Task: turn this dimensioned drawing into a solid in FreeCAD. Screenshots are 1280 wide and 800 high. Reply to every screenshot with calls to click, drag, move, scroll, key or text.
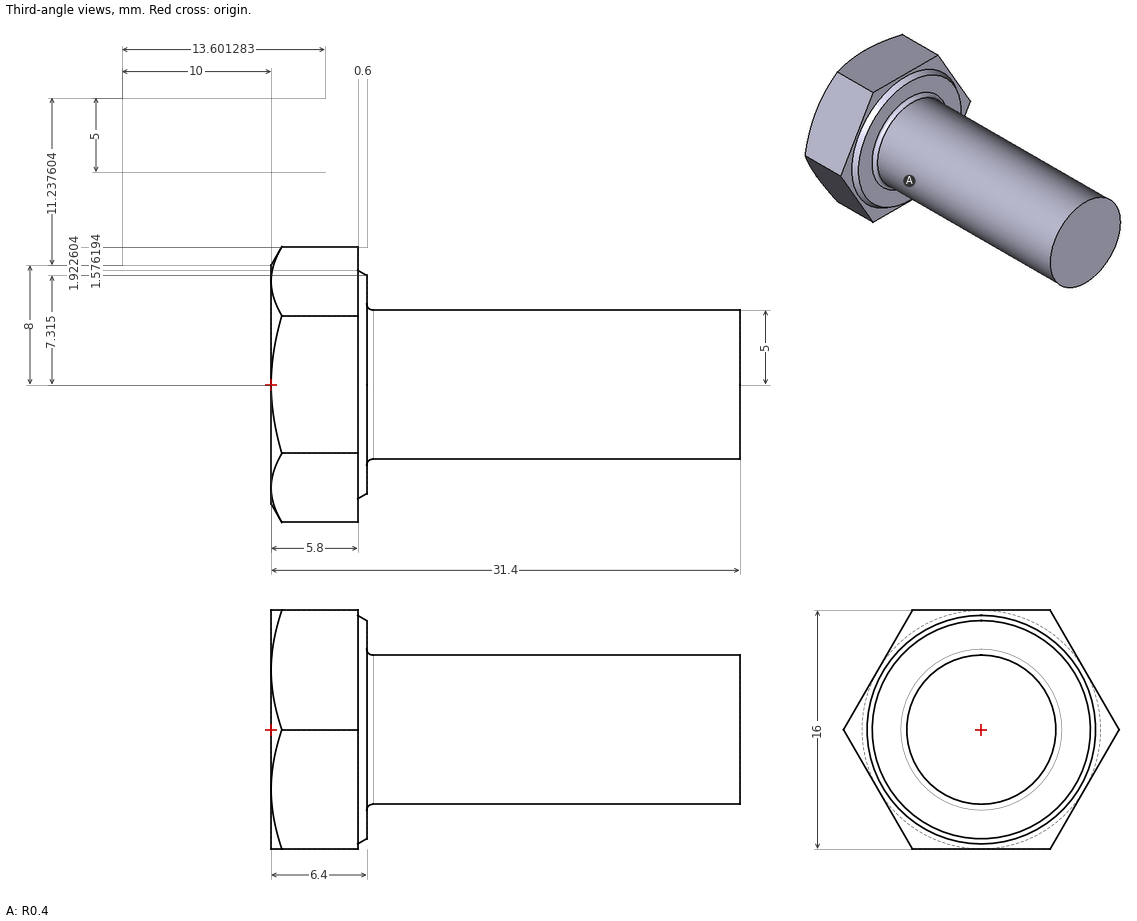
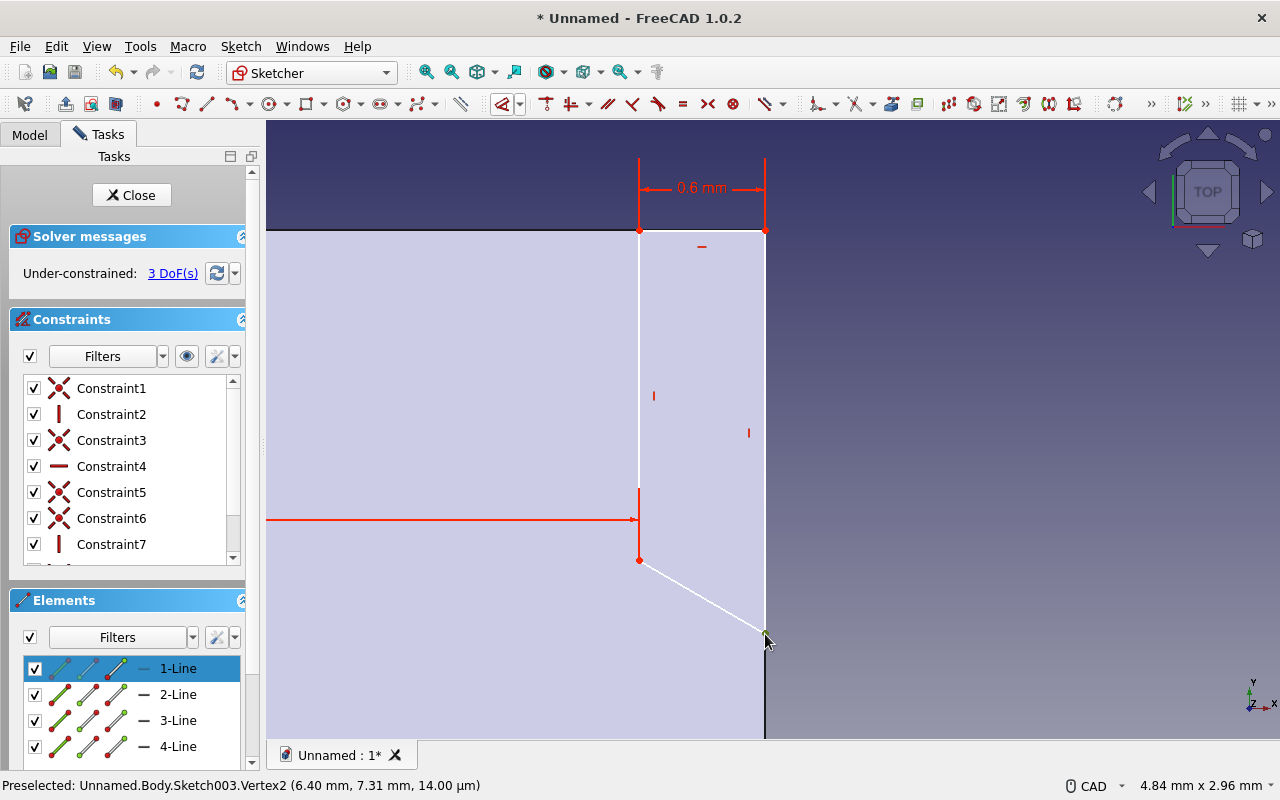
key(i)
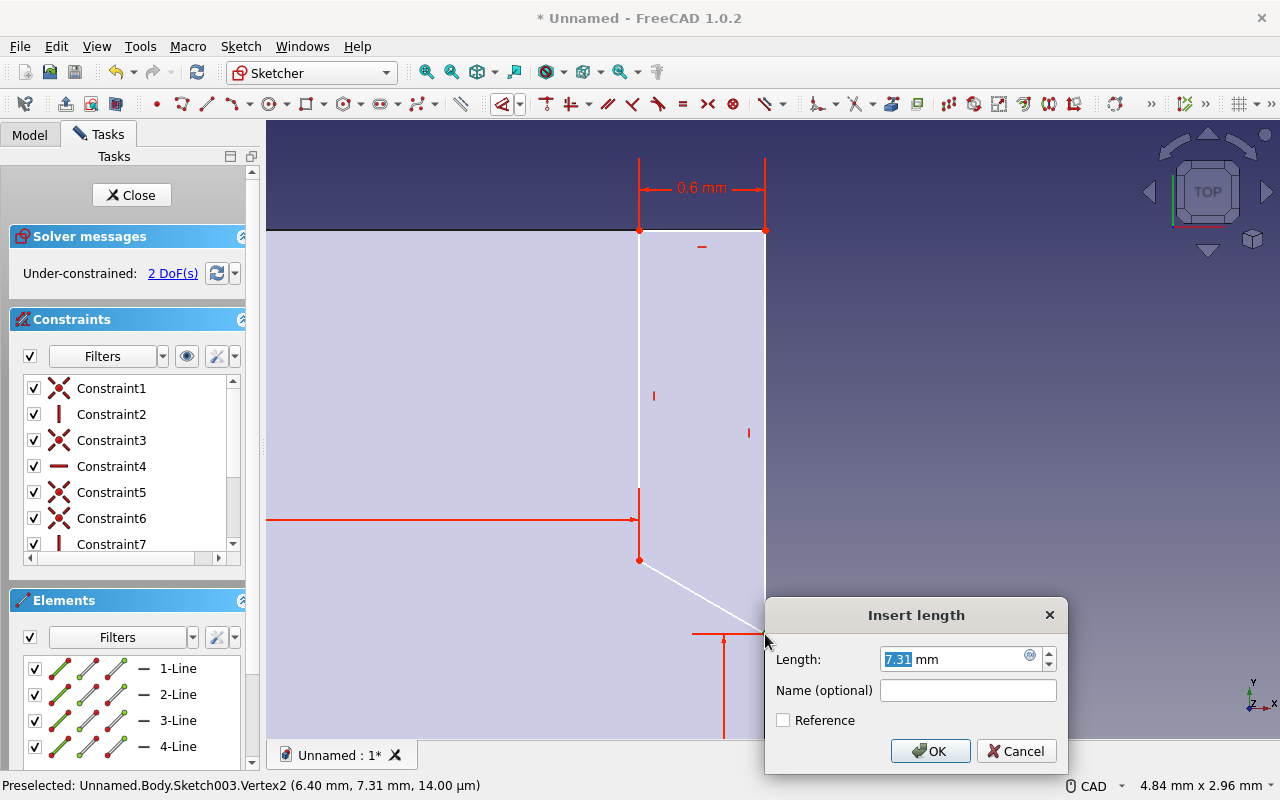
text(7.315)
key(Return)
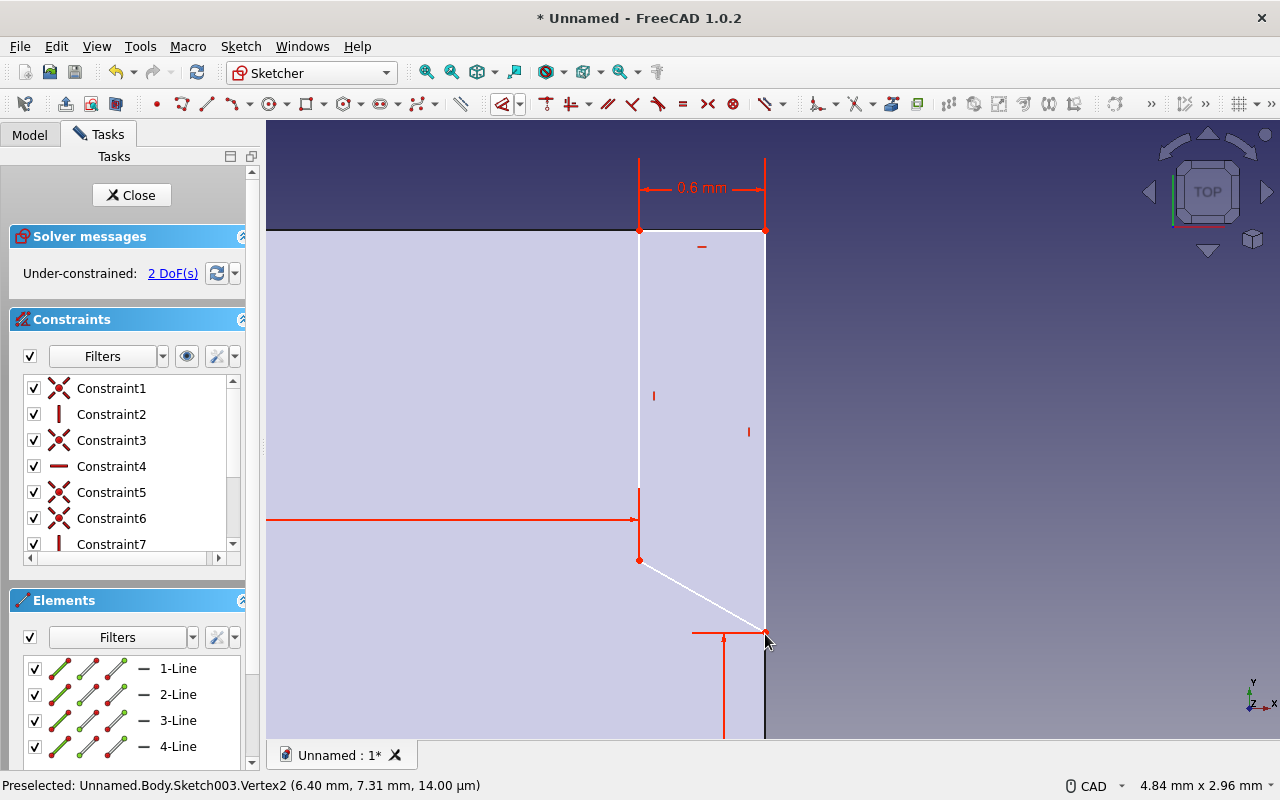
click(765, 512)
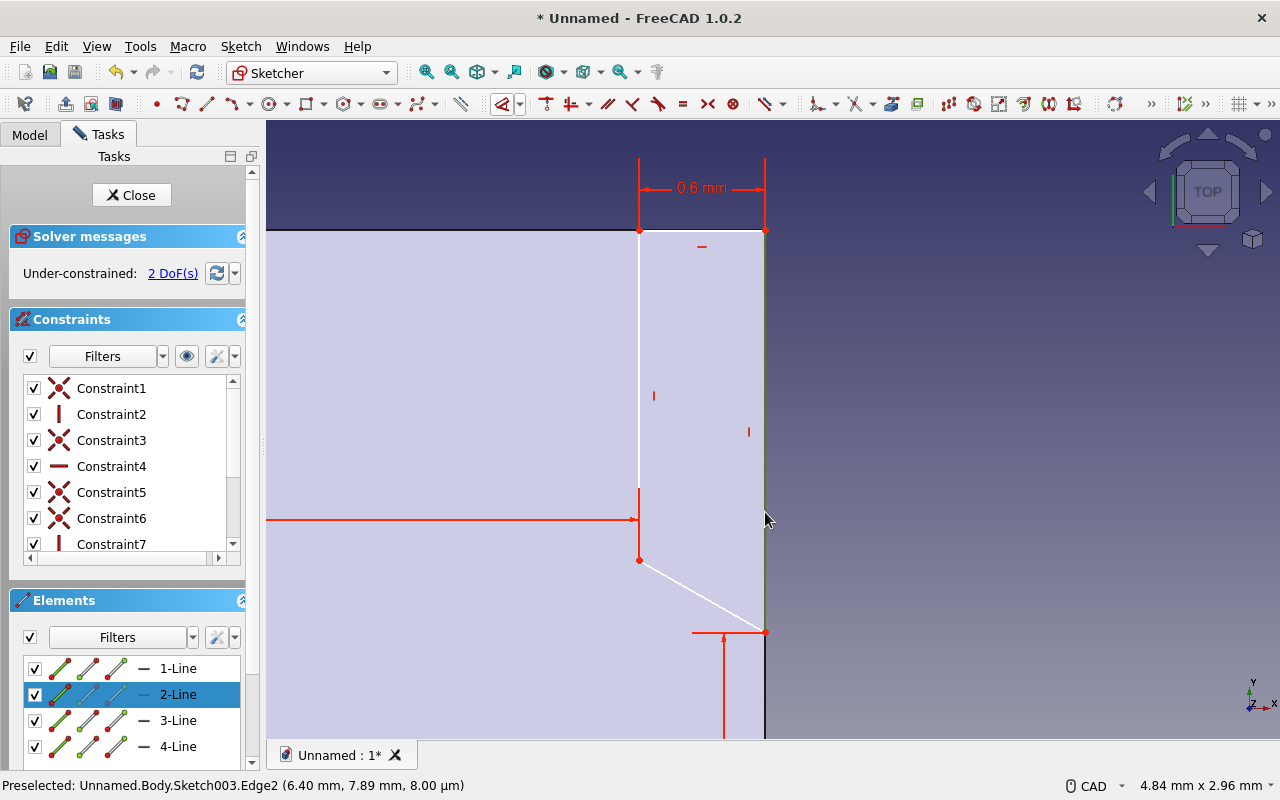
key(i)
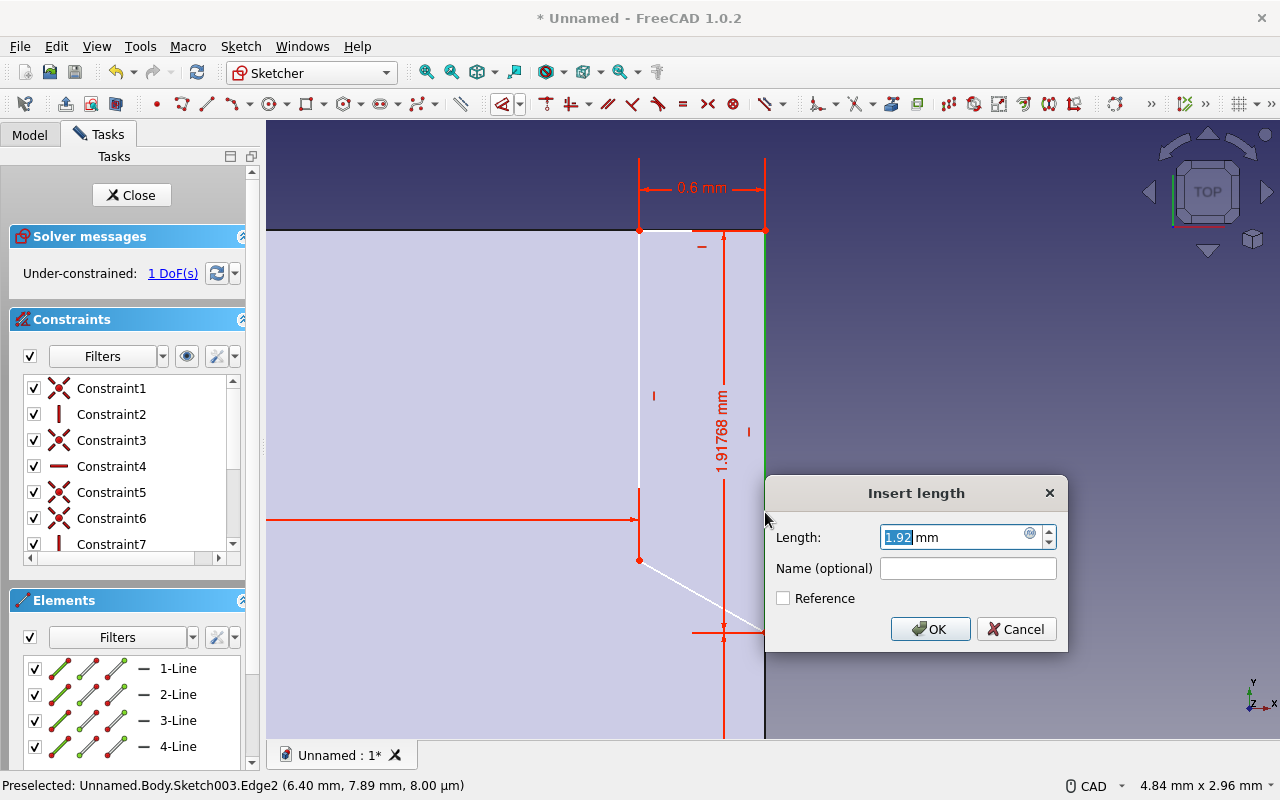
text(1.922604)
key(Return)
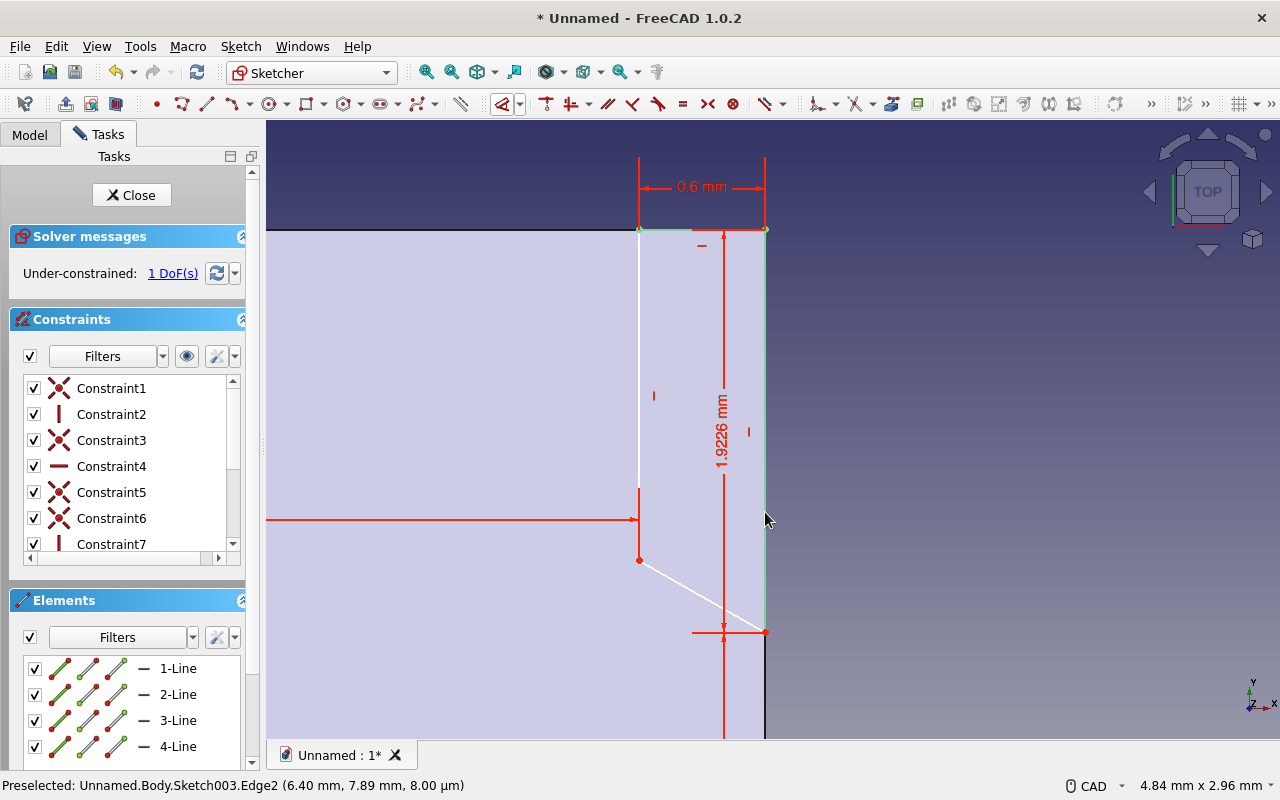
click(639, 329)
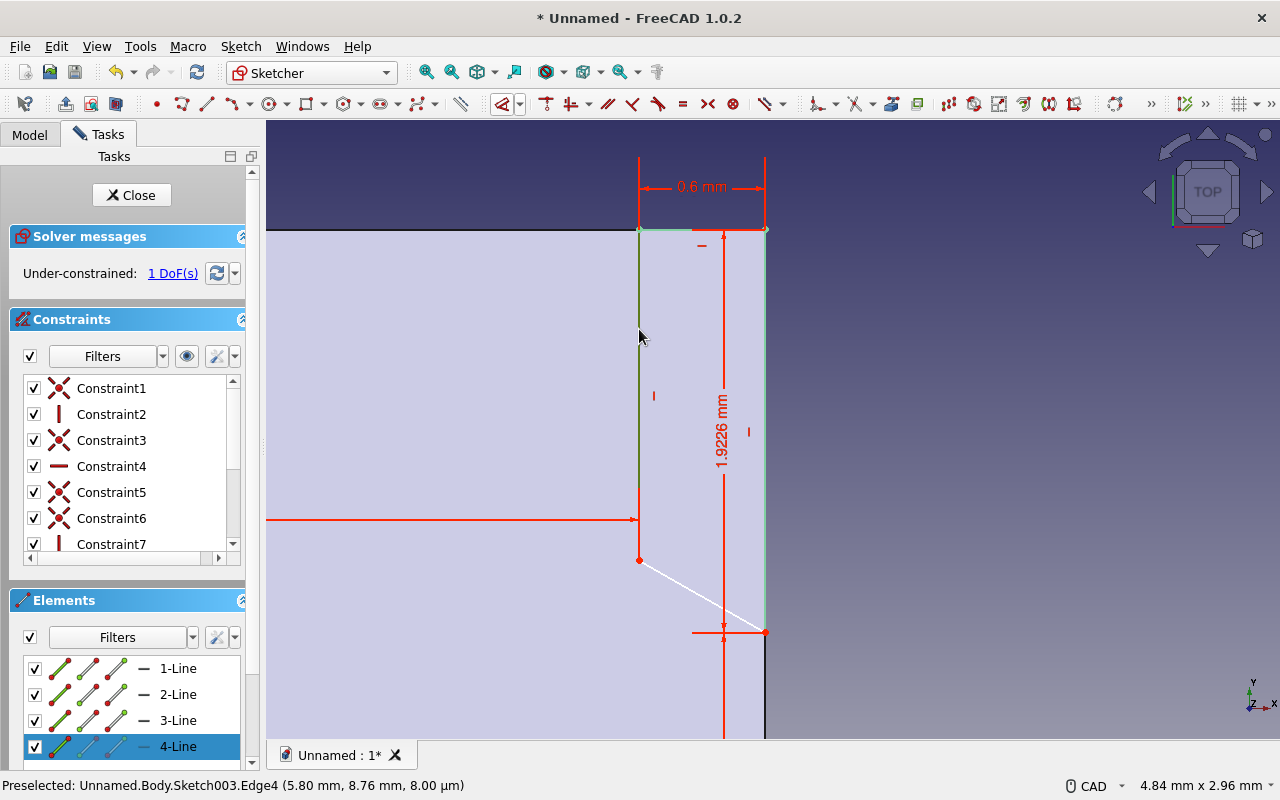
key(i)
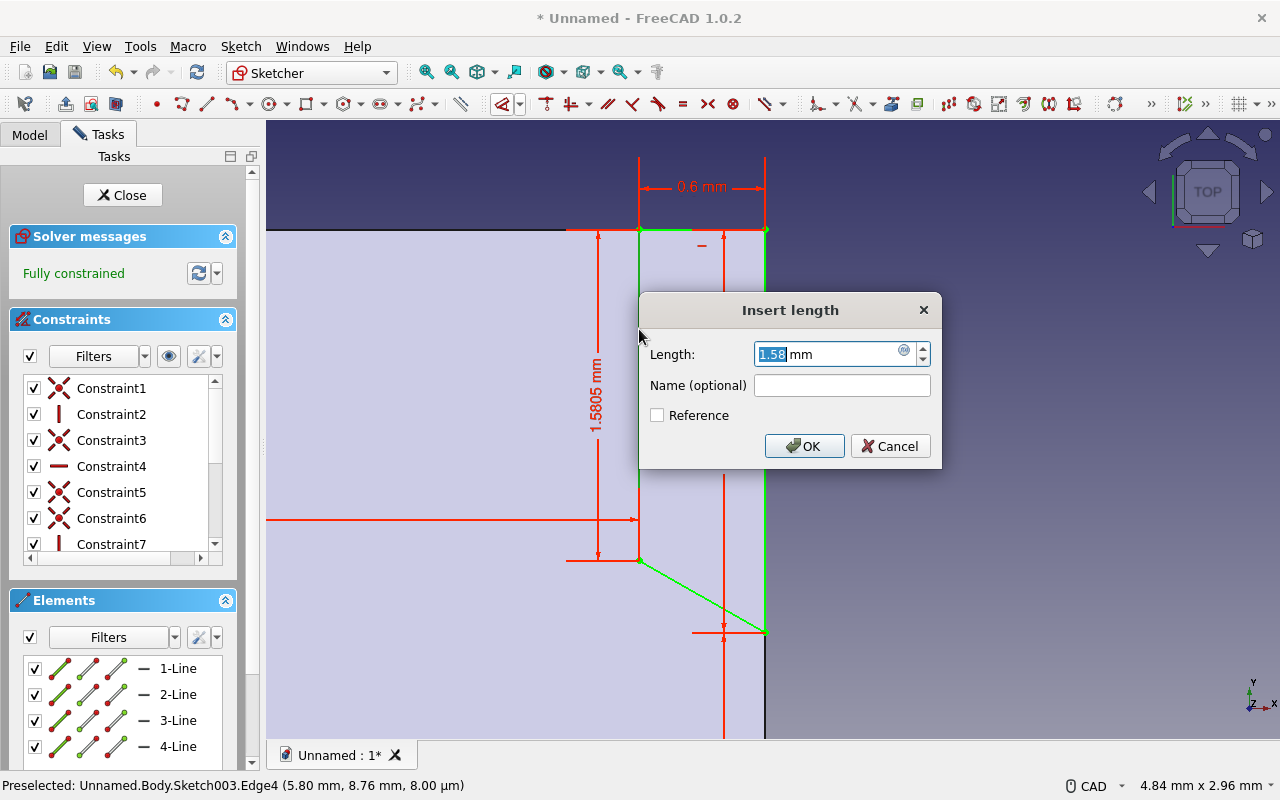
text(1.576194)
key(Return)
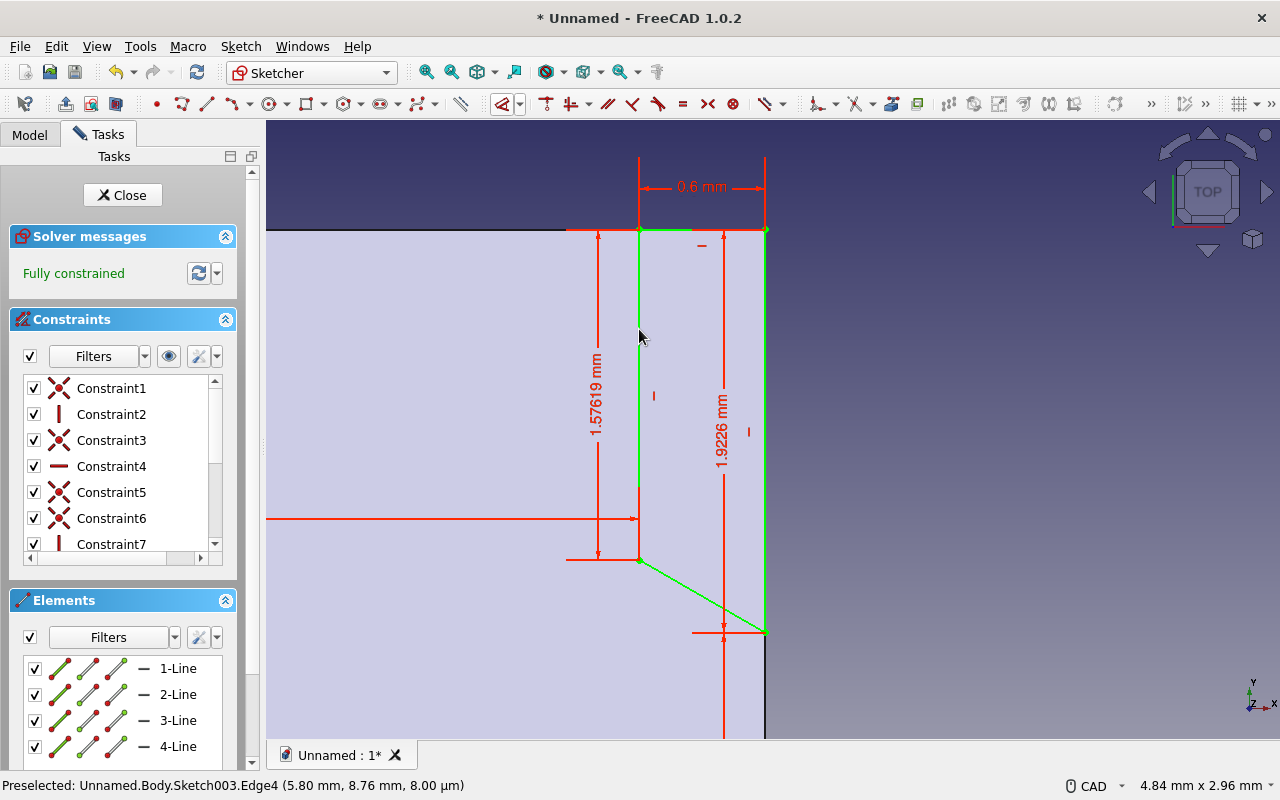
click(123, 195)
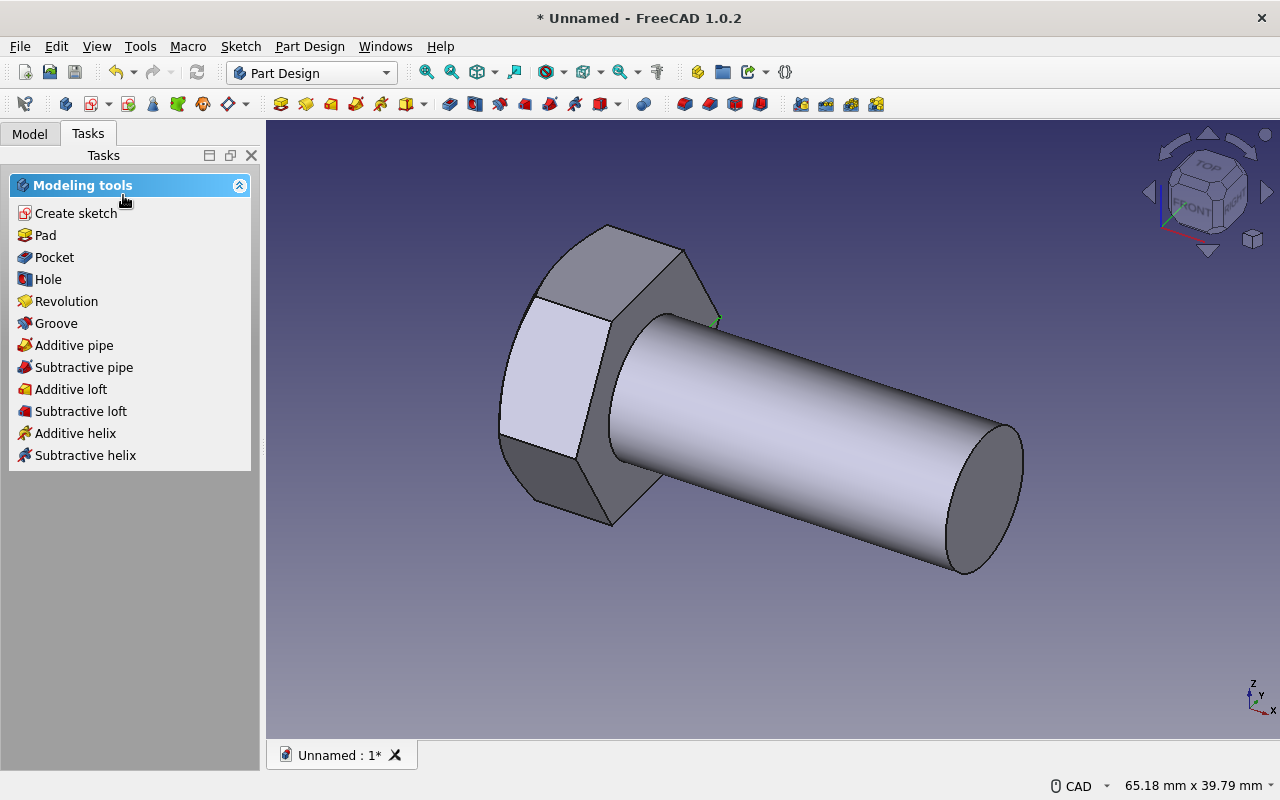
click(500, 104)